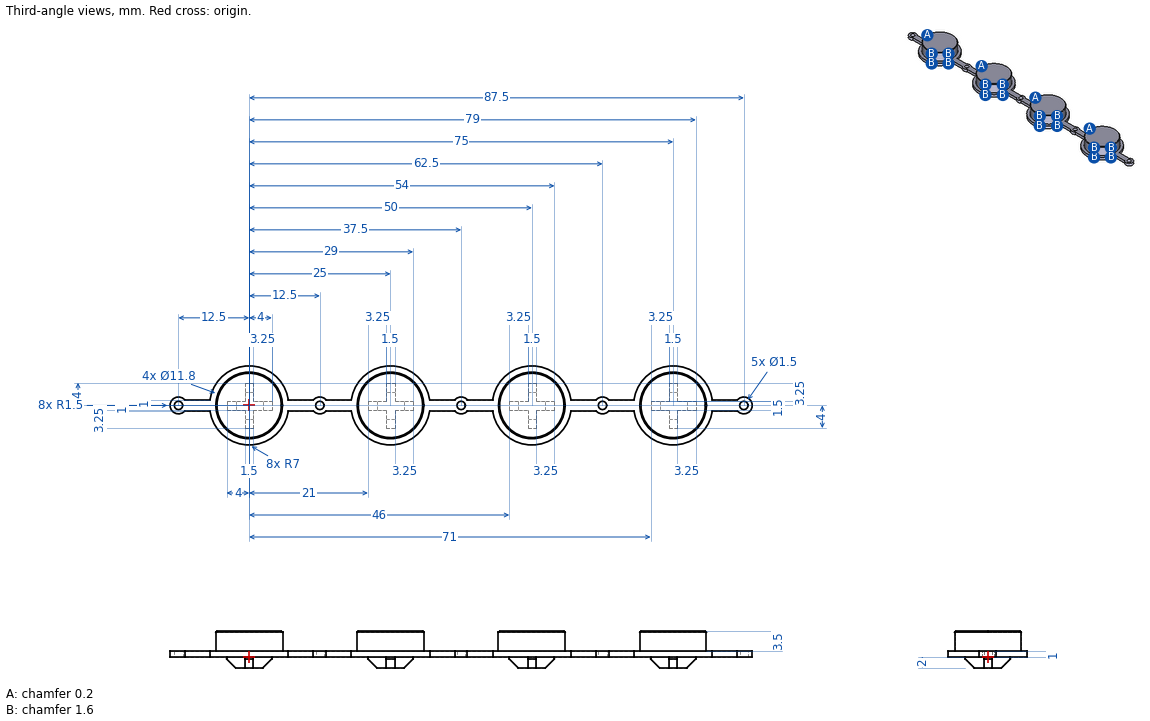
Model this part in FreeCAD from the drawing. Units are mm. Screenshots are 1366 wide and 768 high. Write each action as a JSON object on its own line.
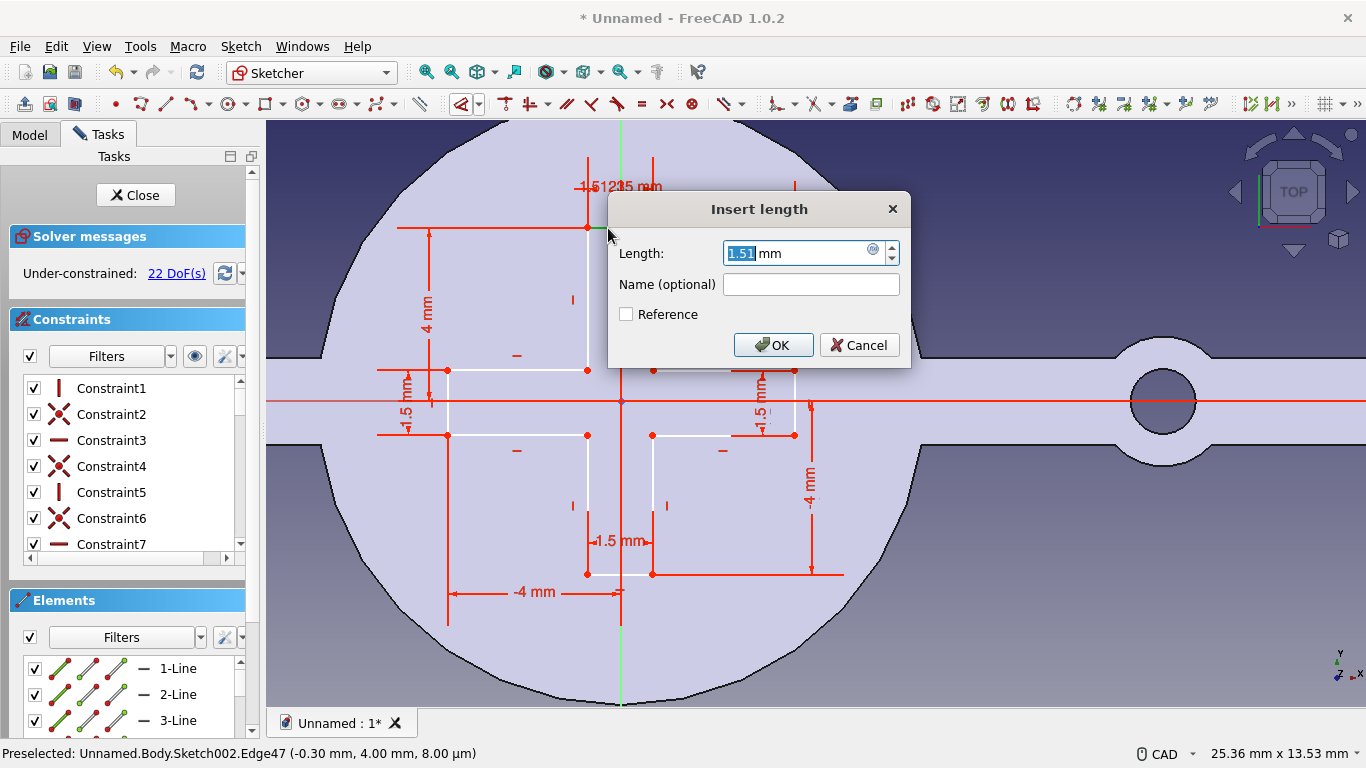
{"action": "type", "text": "1.5"}
{"action": "key", "text": "Return"}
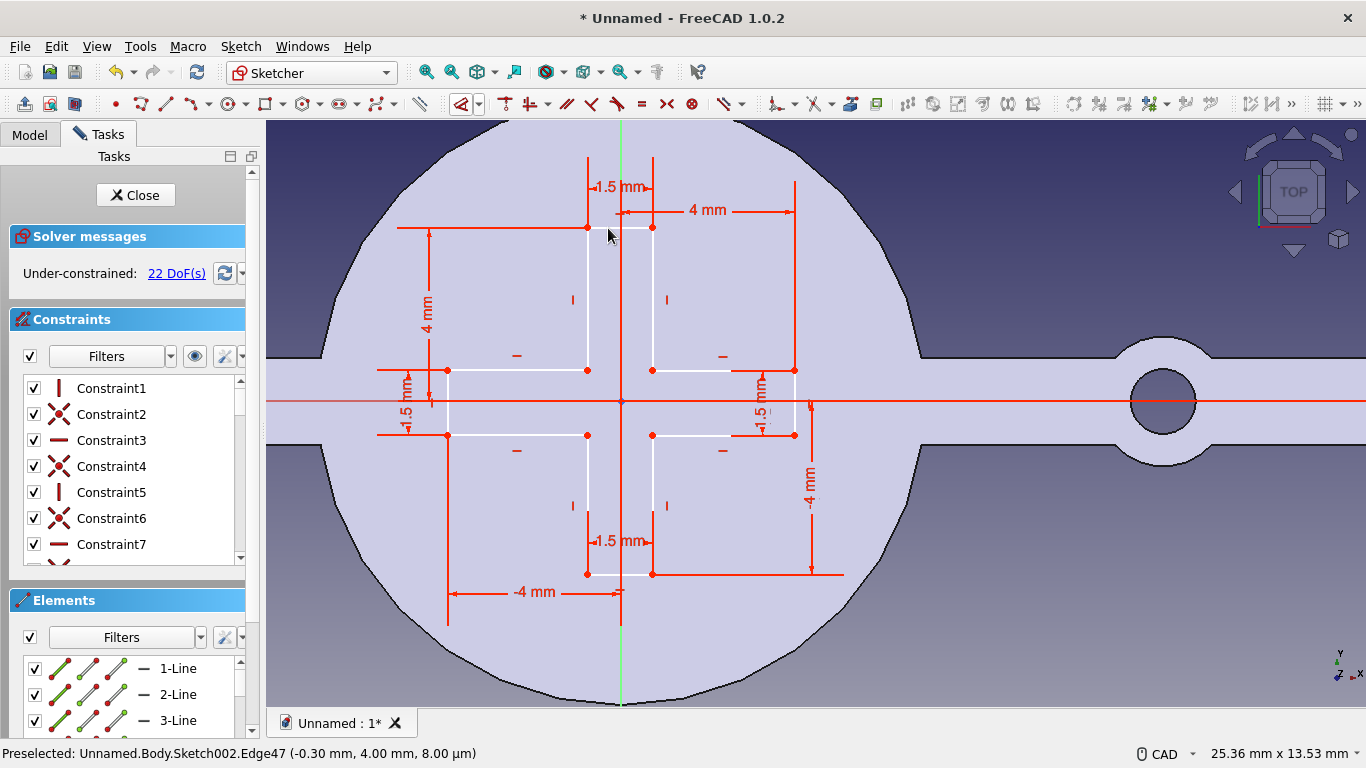
{"action": "scroll", "coordinate": [450, 416], "scroll_direction": "down", "scroll_amount": 9}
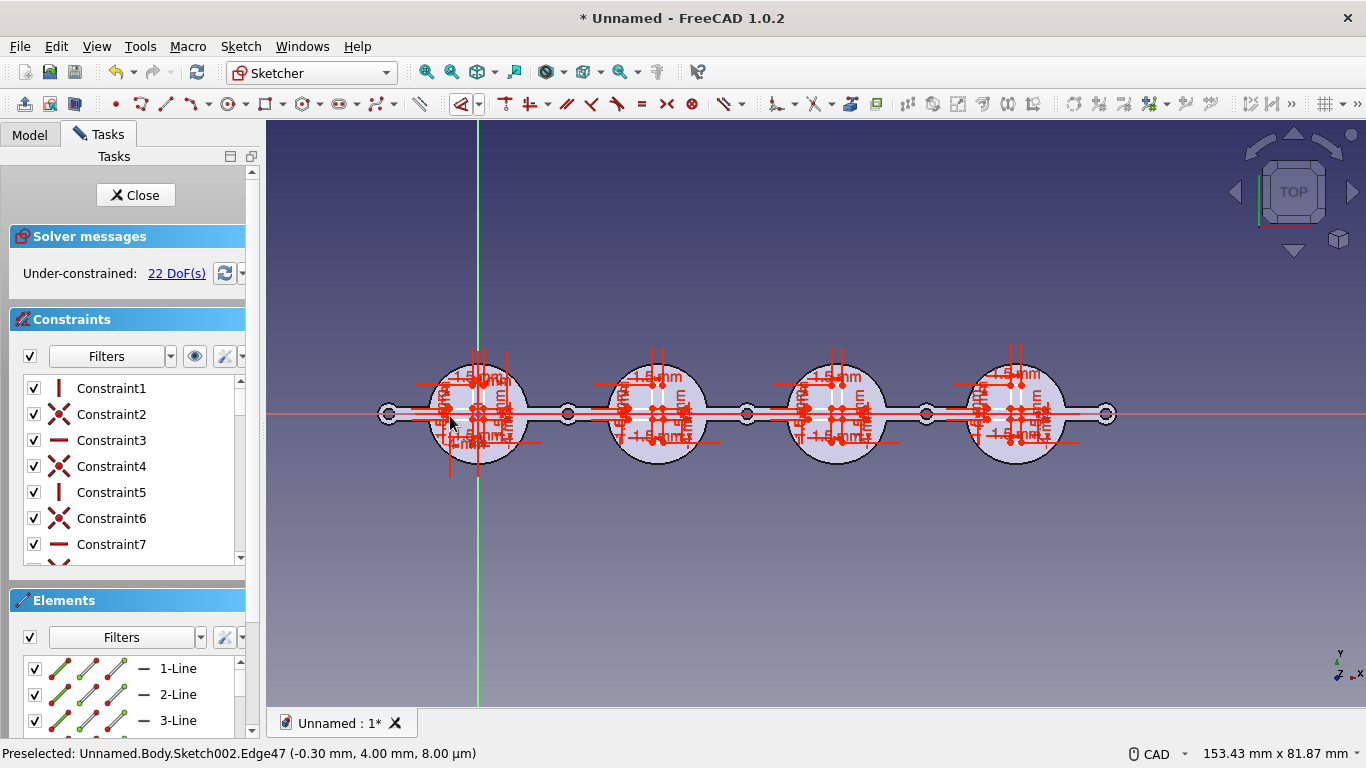
{"action": "left_click", "coordinate": [988, 420]}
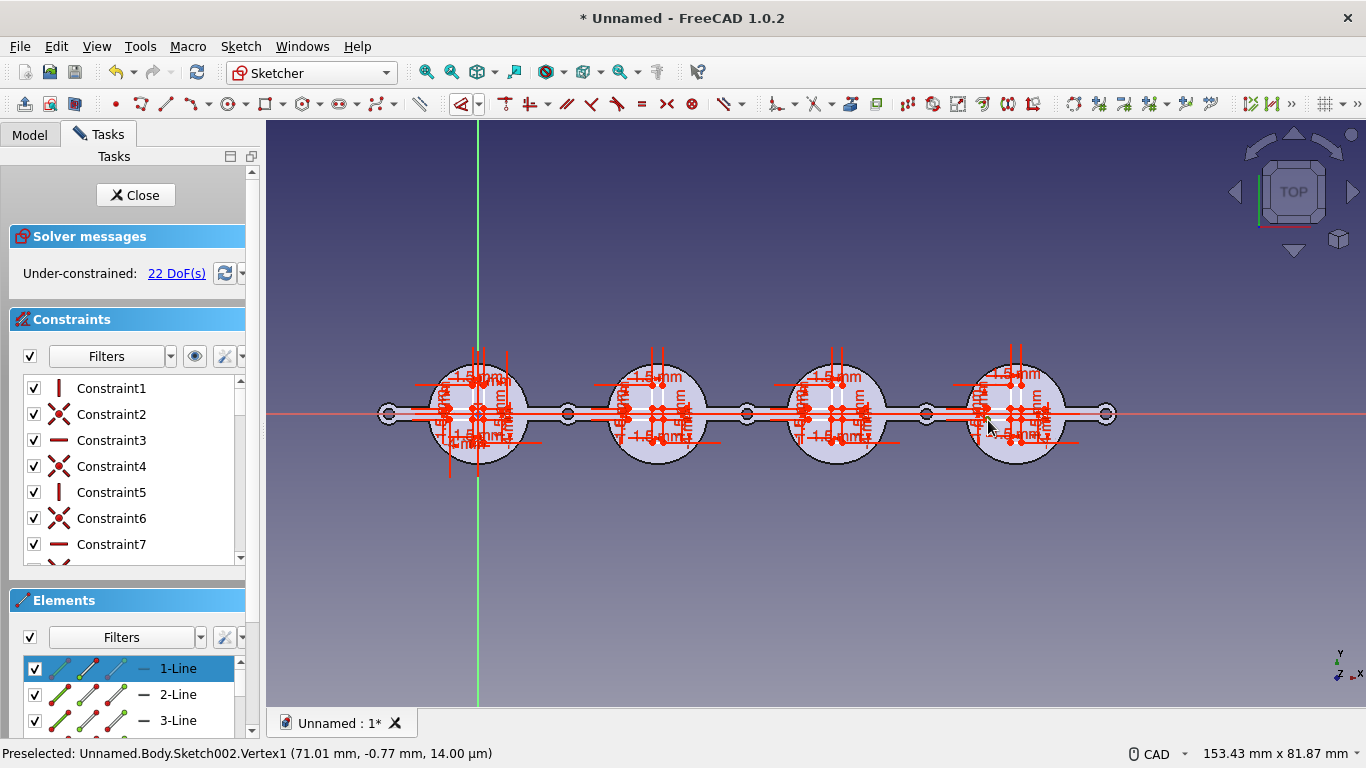
{"action": "key", "text": "l"}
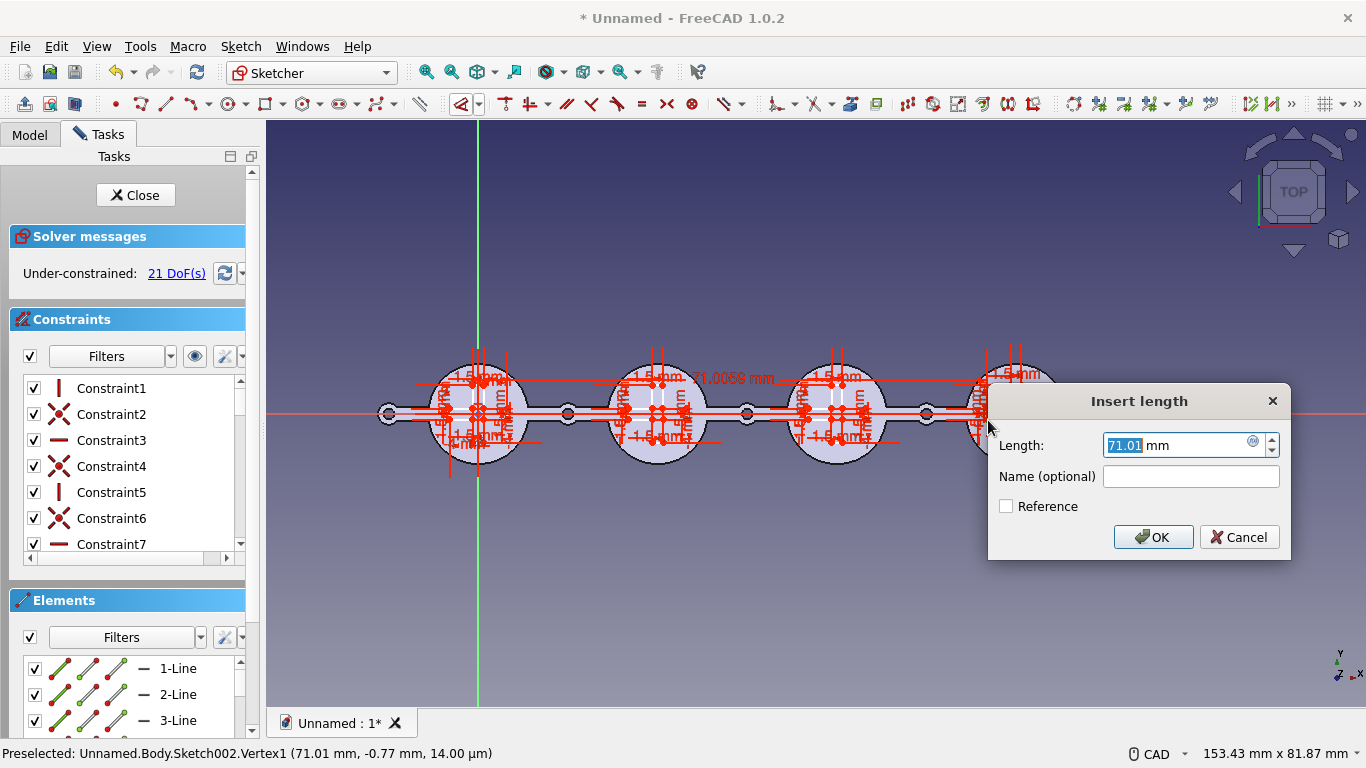
{"action": "type", "text": "71"}
{"action": "key", "text": "Return"}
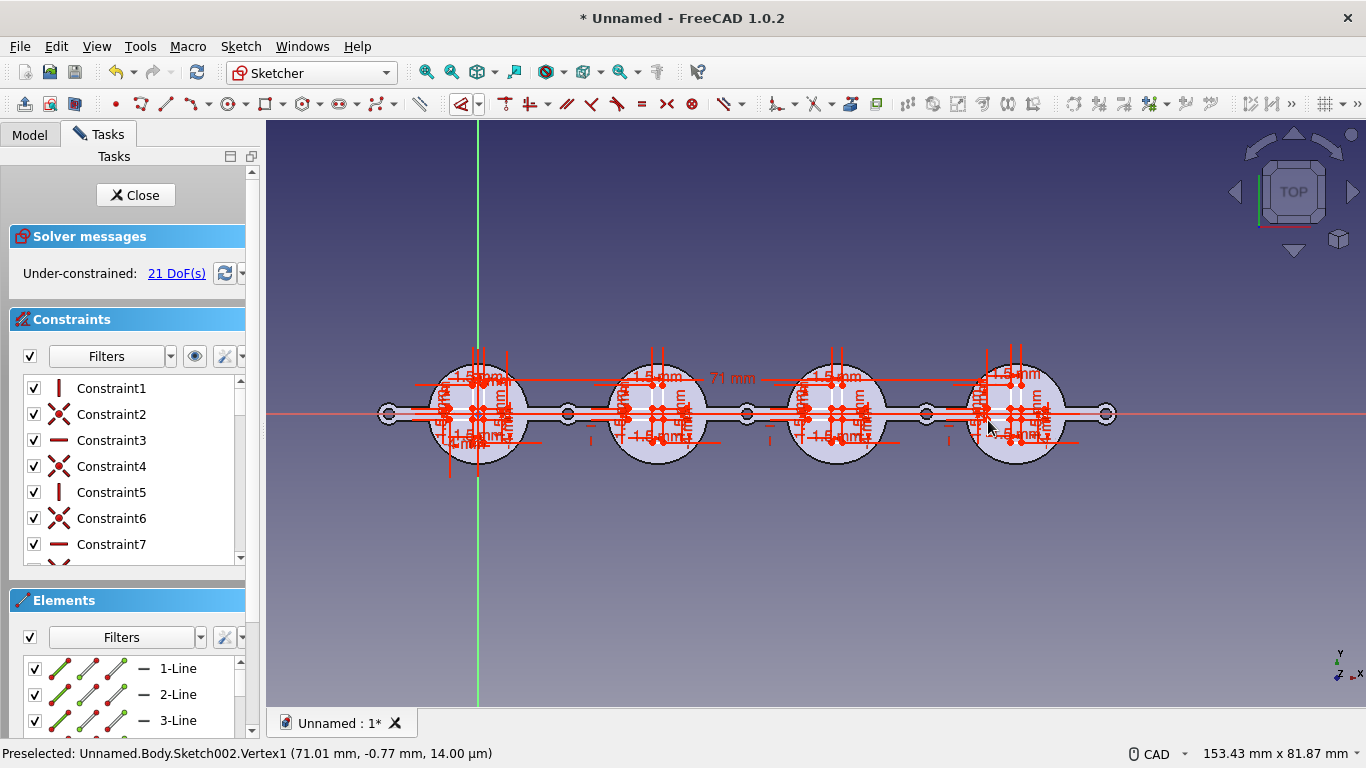
{"action": "left_click", "coordinate": [1045, 409]}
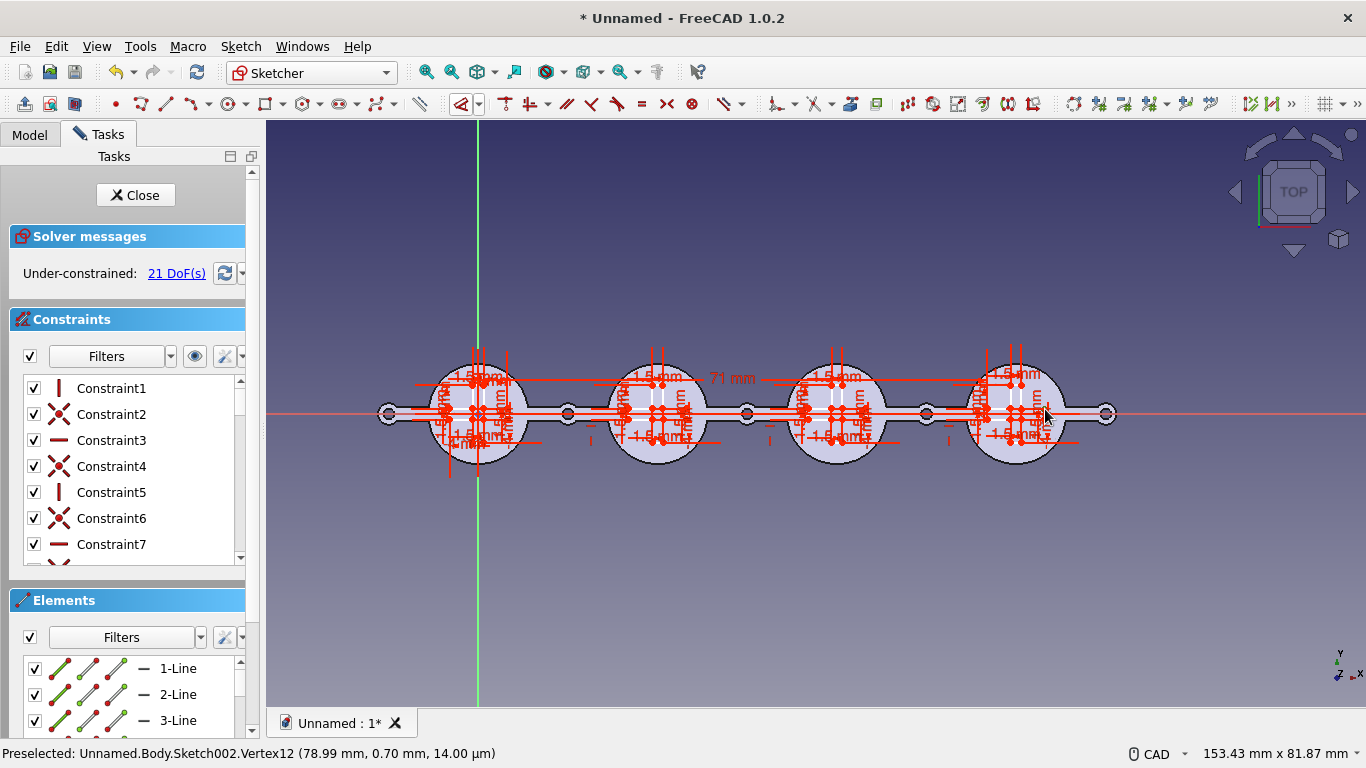
{"action": "key", "text": "l"}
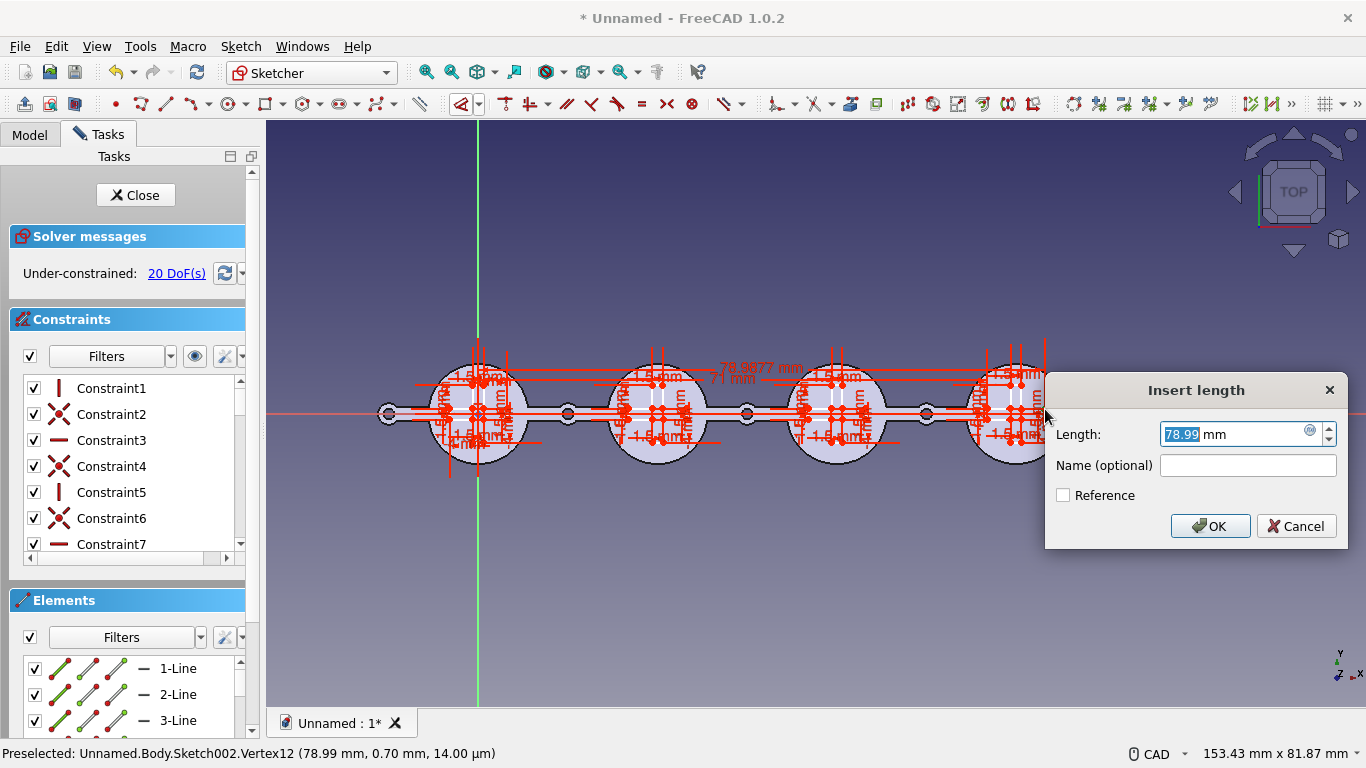
{"action": "type", "text": "79"}
{"action": "key", "text": "Return"}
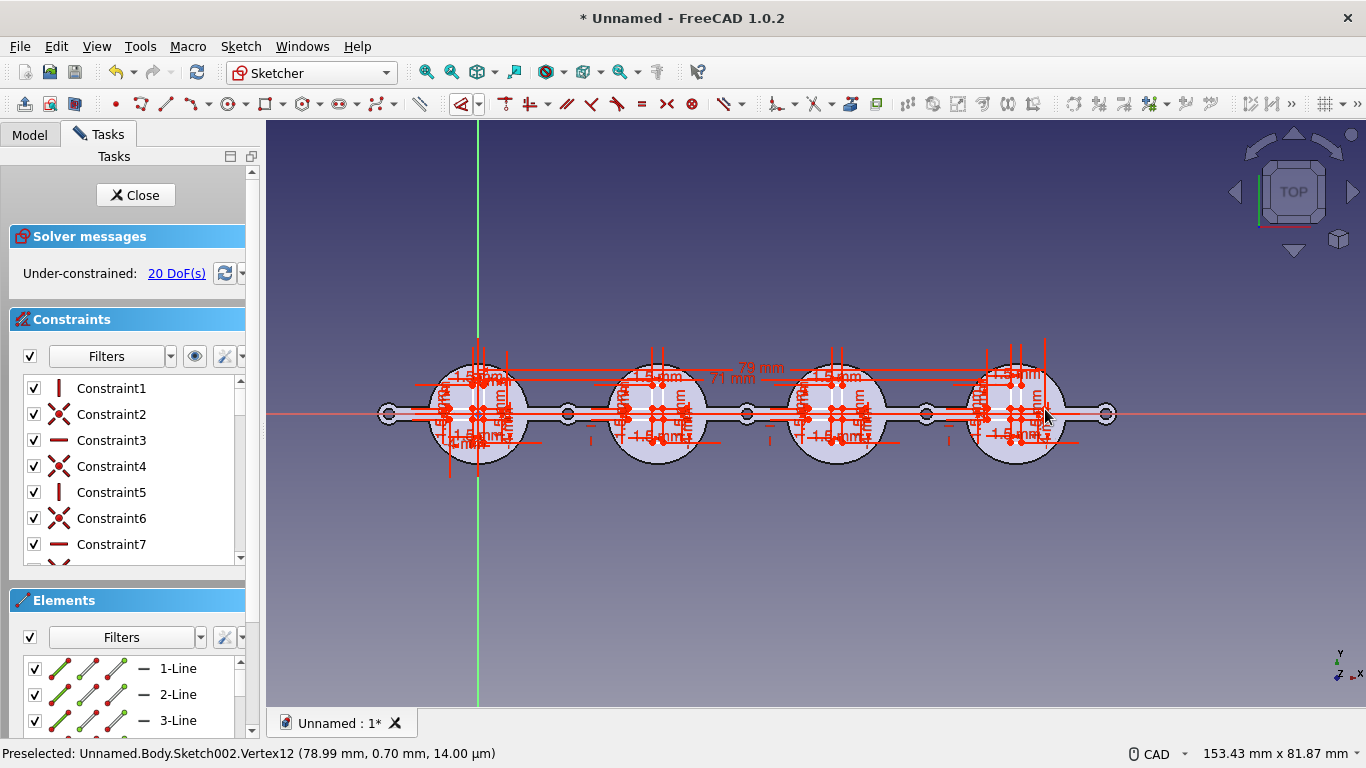
{"action": "left_click", "coordinate": [808, 420]}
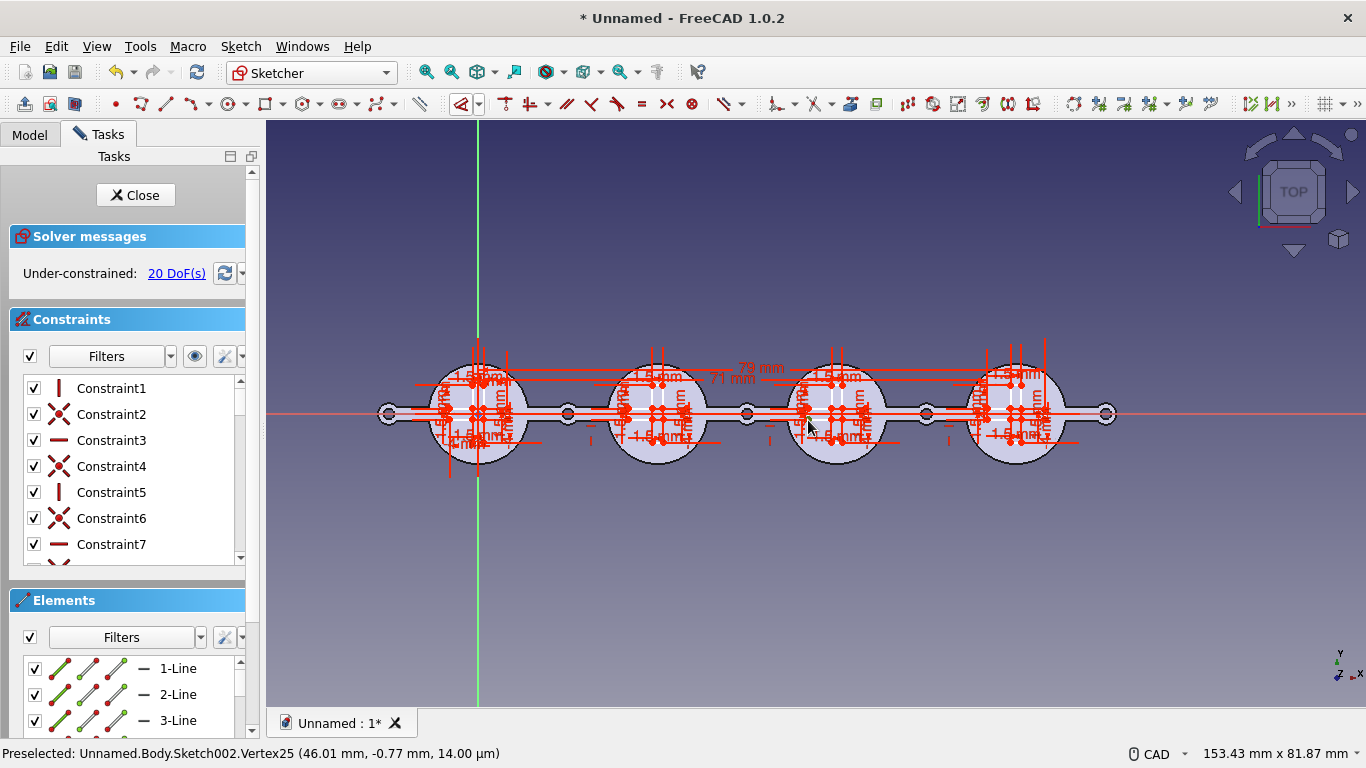
{"action": "left_click", "coordinate": [478, 104]}